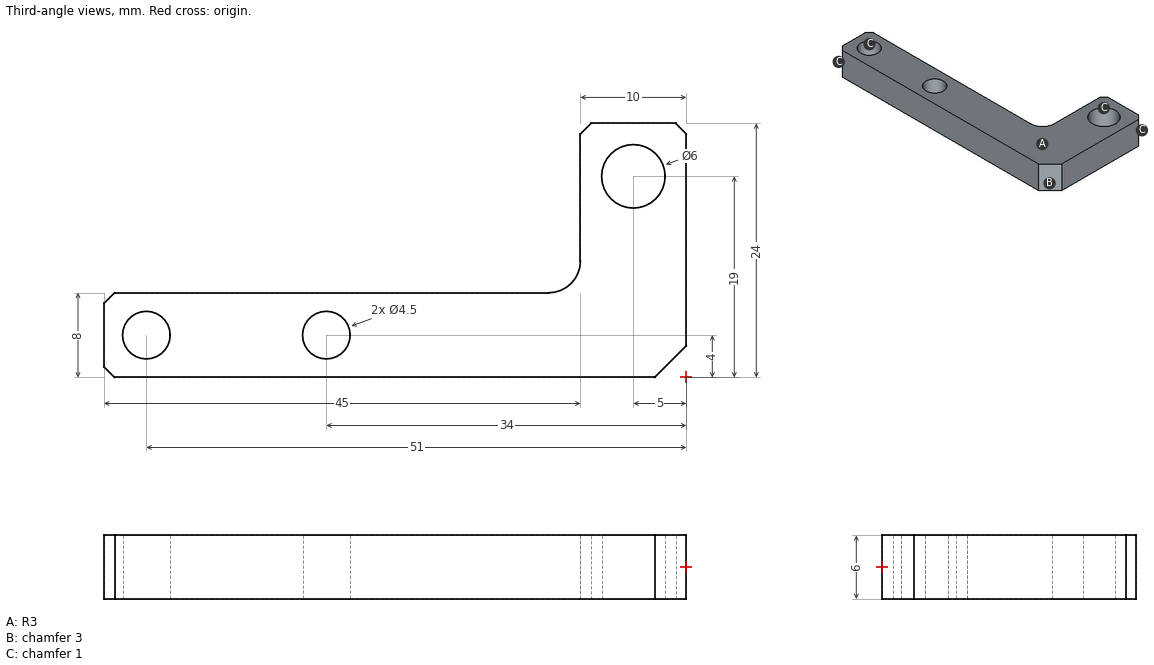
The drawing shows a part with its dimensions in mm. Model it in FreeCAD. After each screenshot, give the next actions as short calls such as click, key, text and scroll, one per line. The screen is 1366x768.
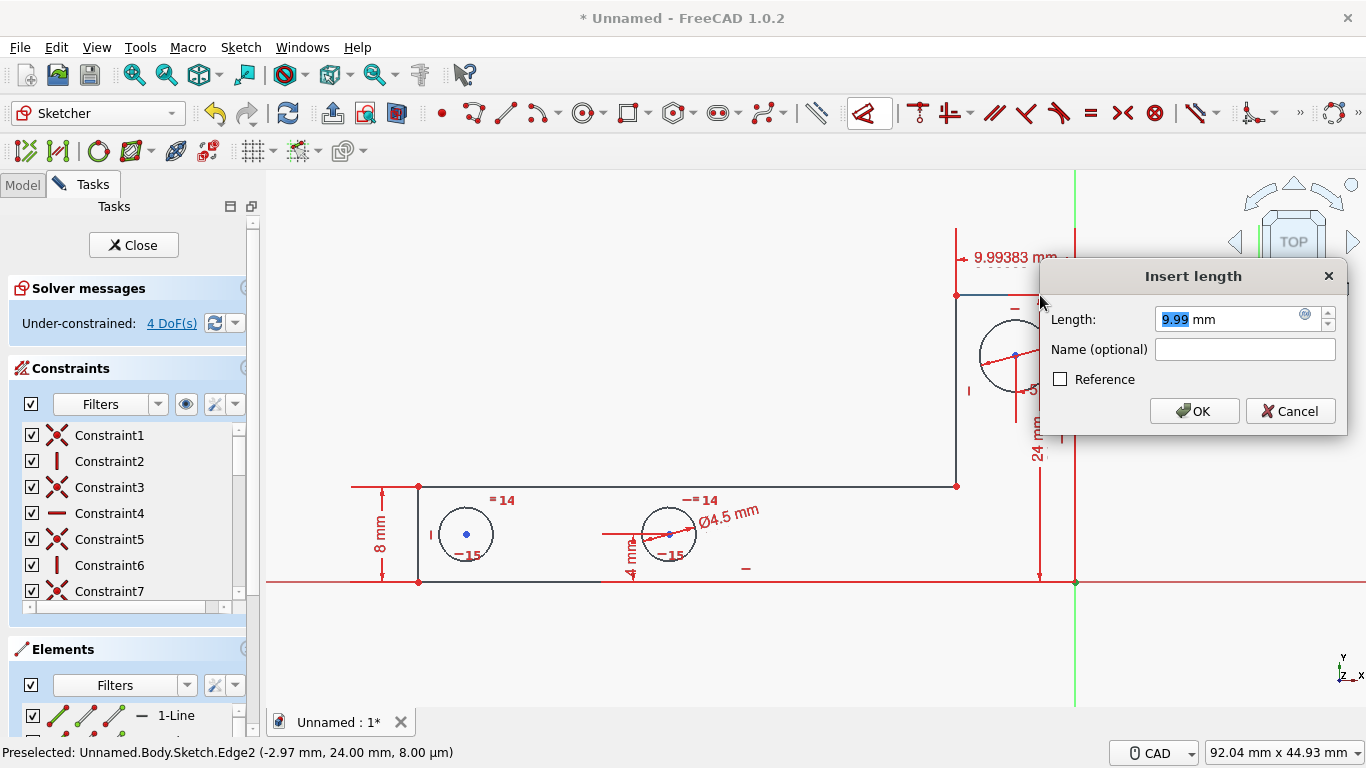
text(10)
key(Return)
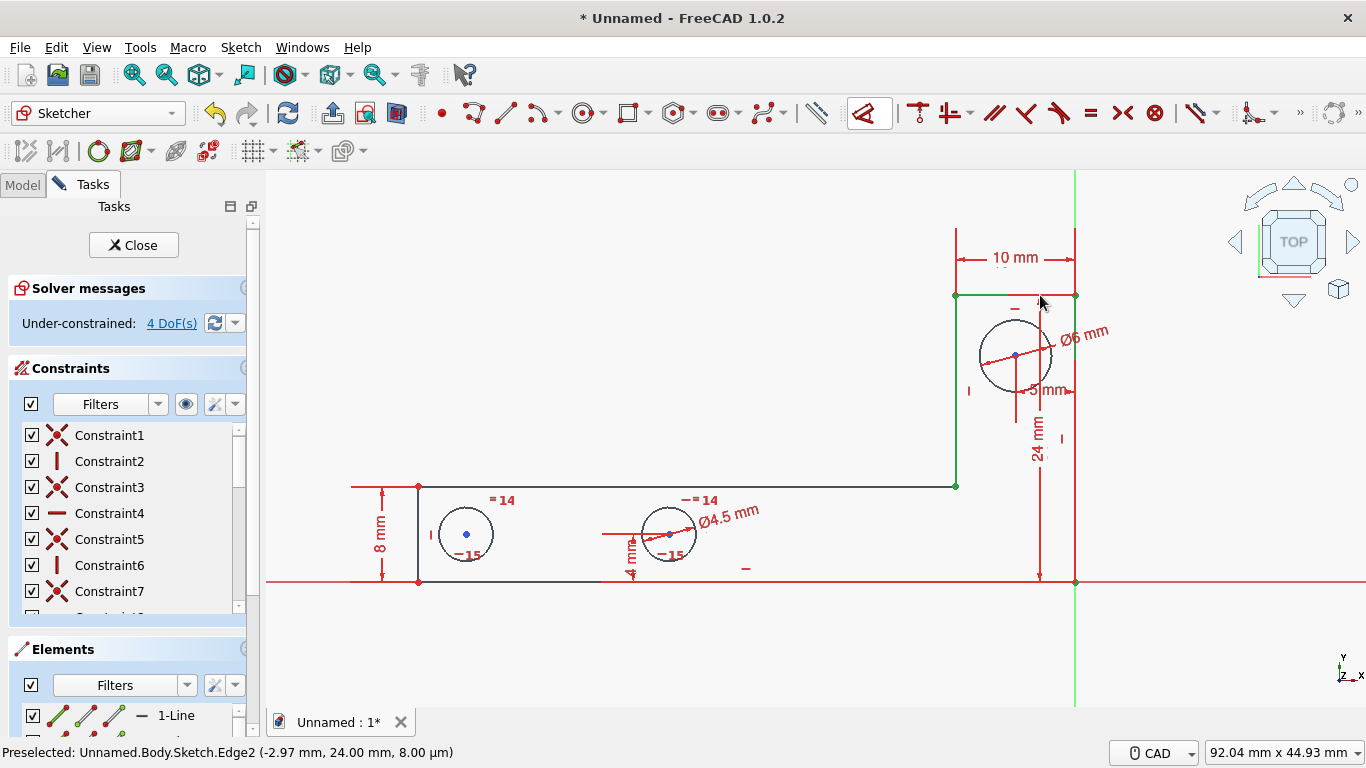
click(795, 487)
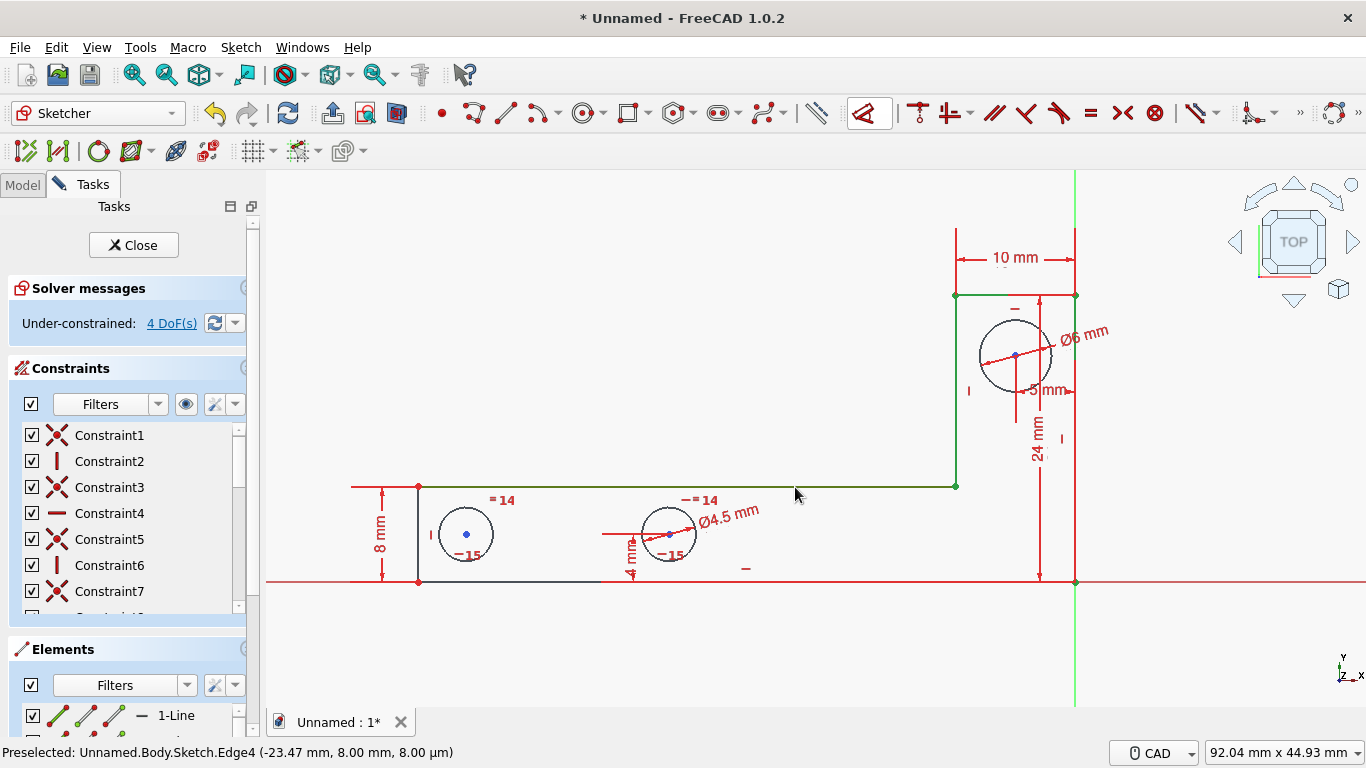
key(l)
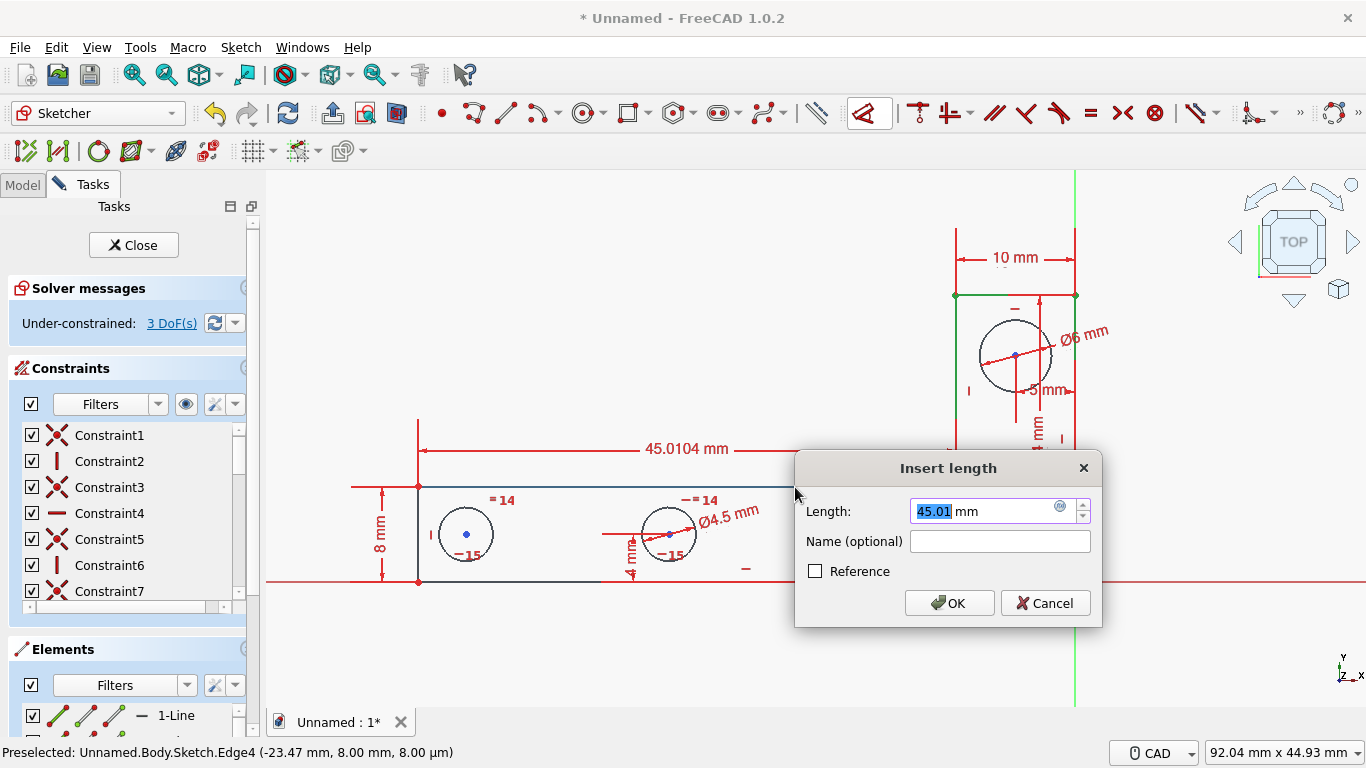
text(45)
key(Return)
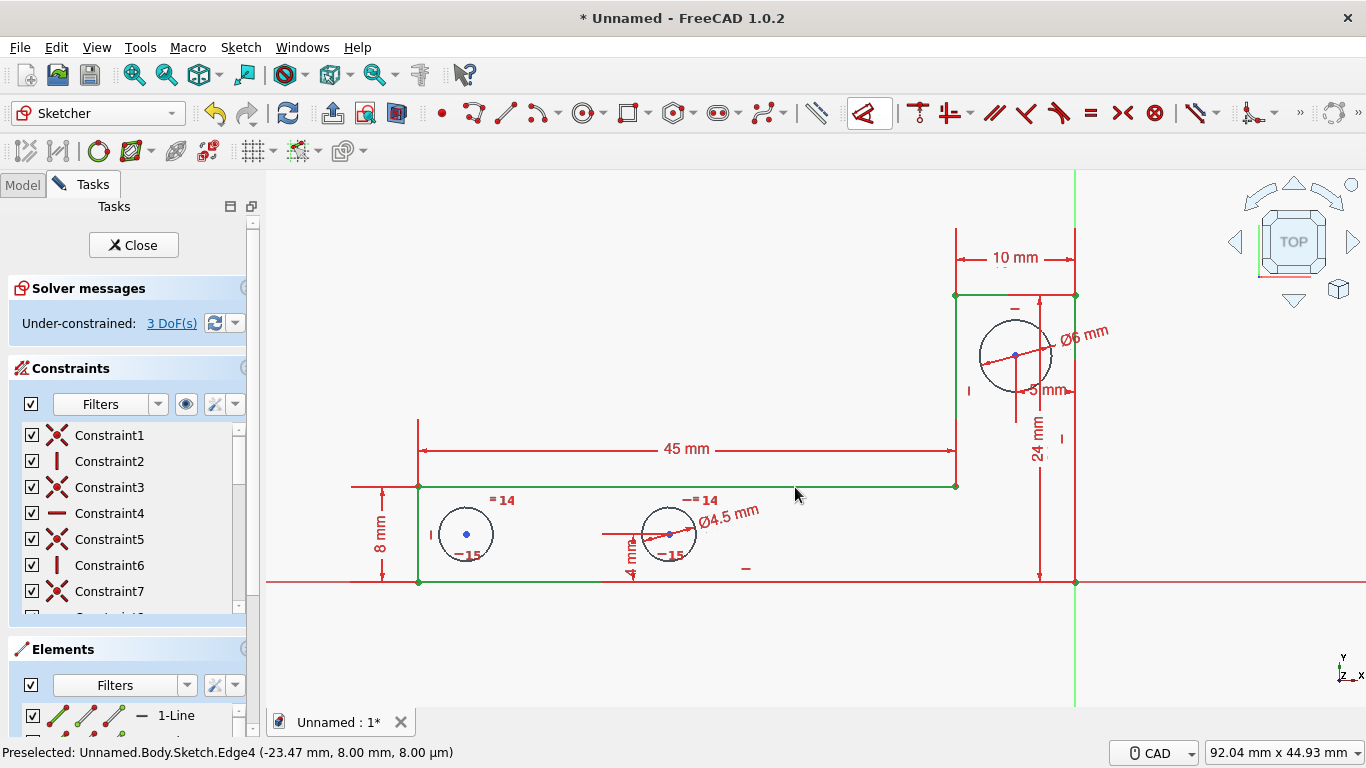
click(669, 534)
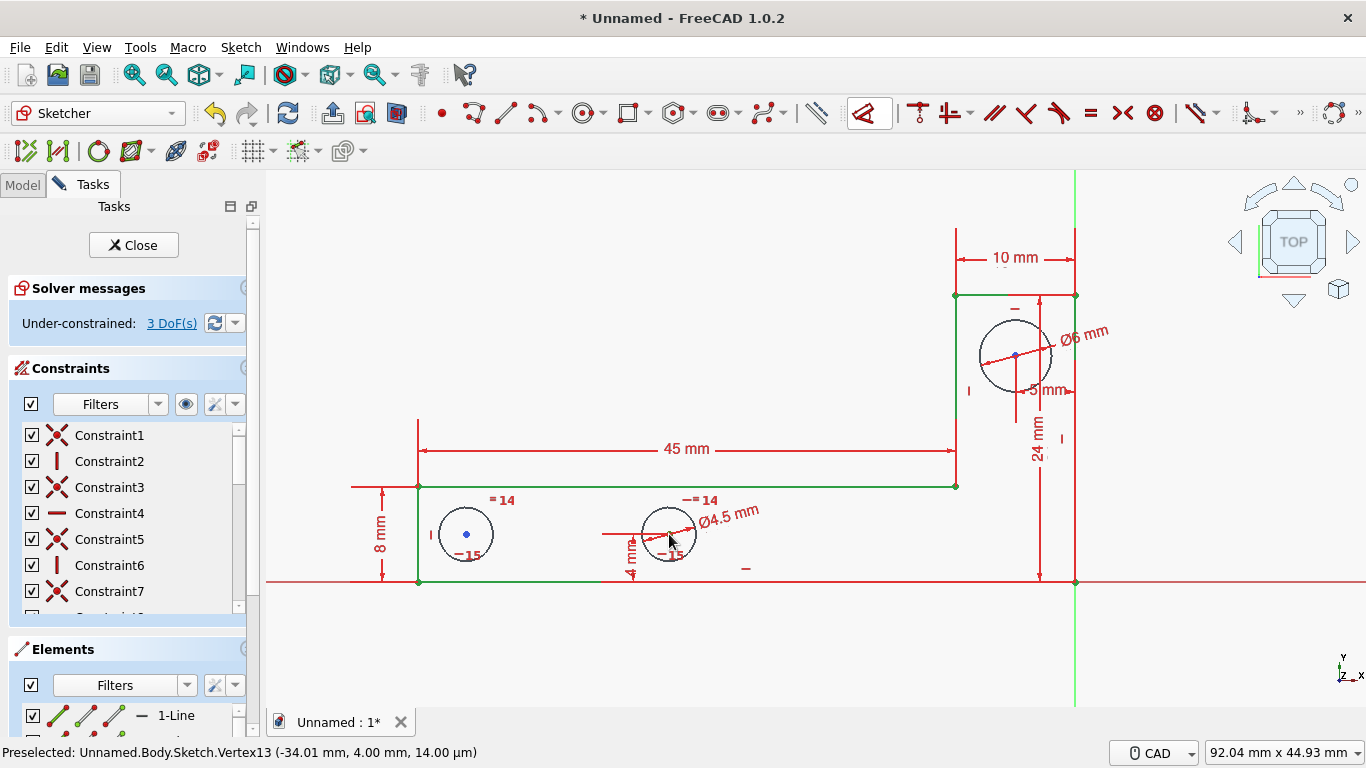
key(l)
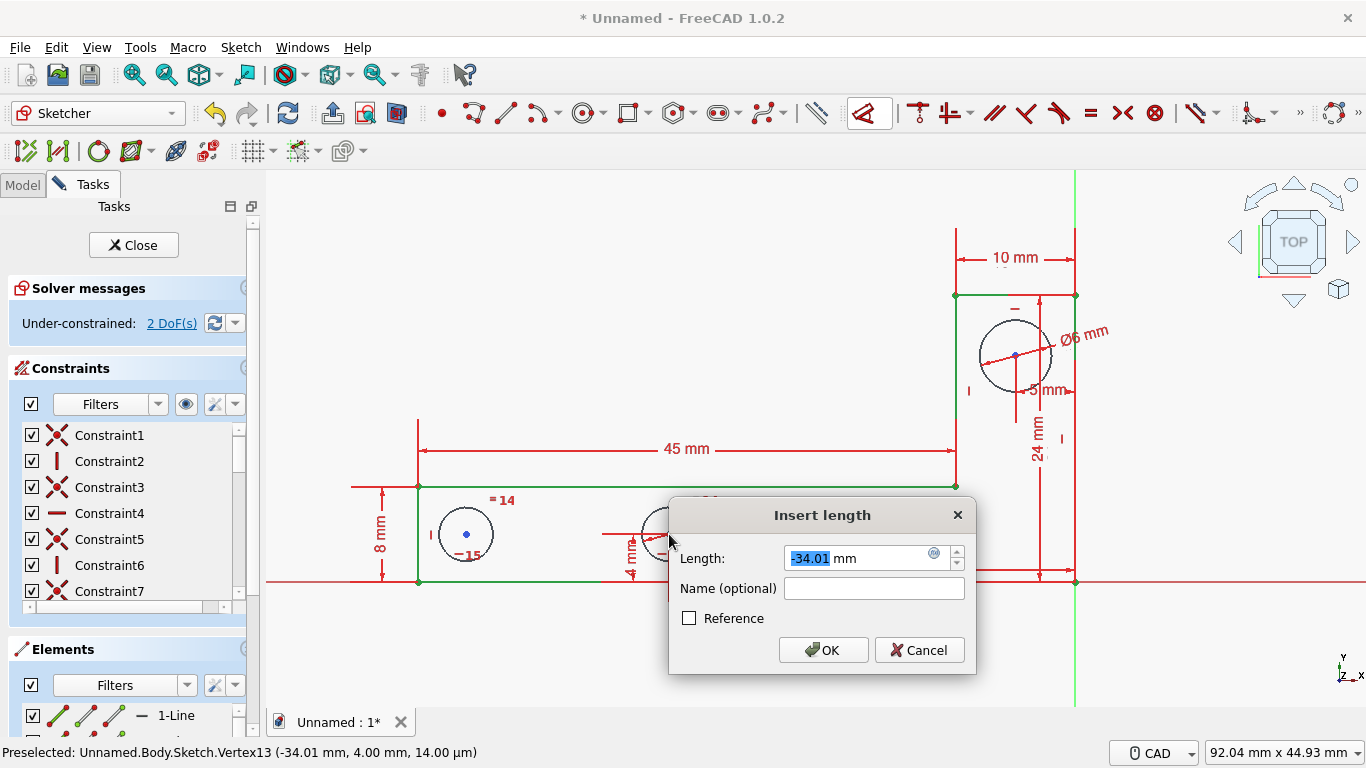
text(-34)
key(Return)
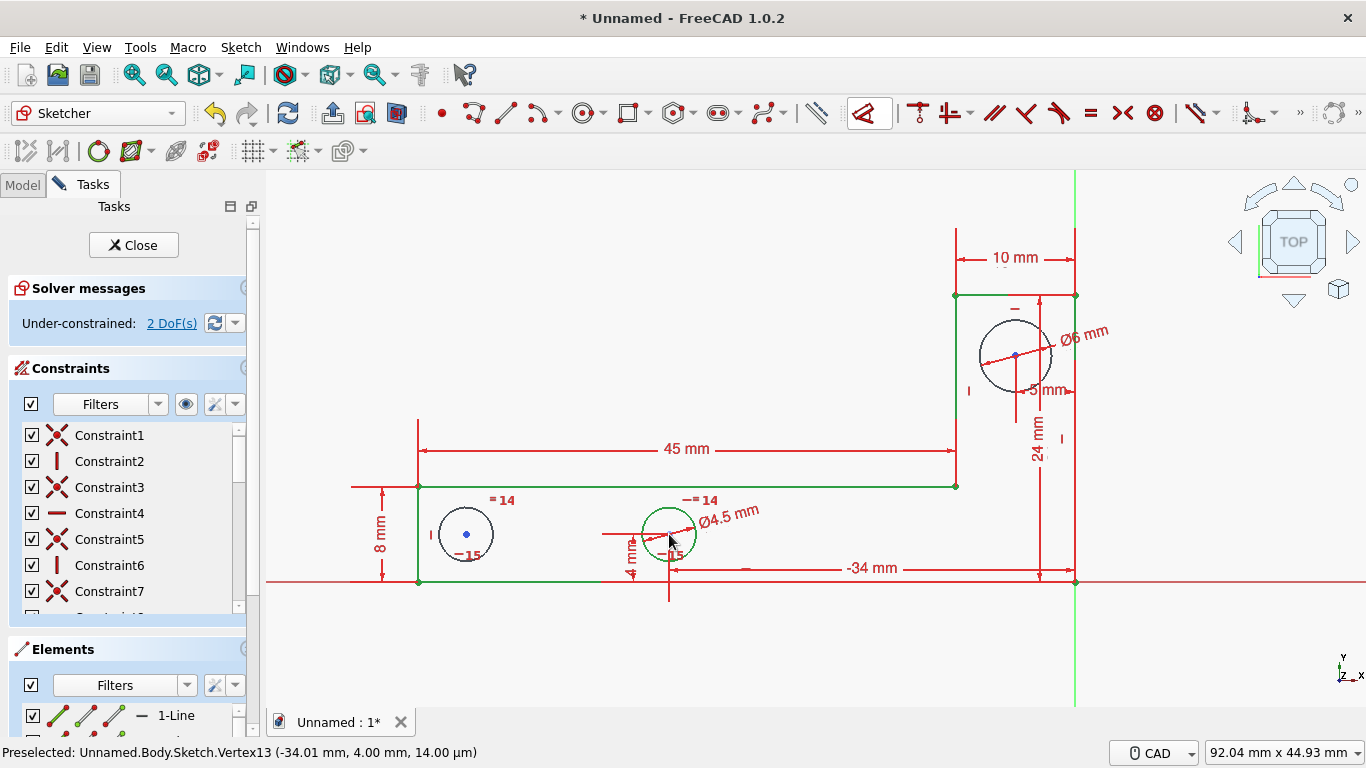
click(466, 534)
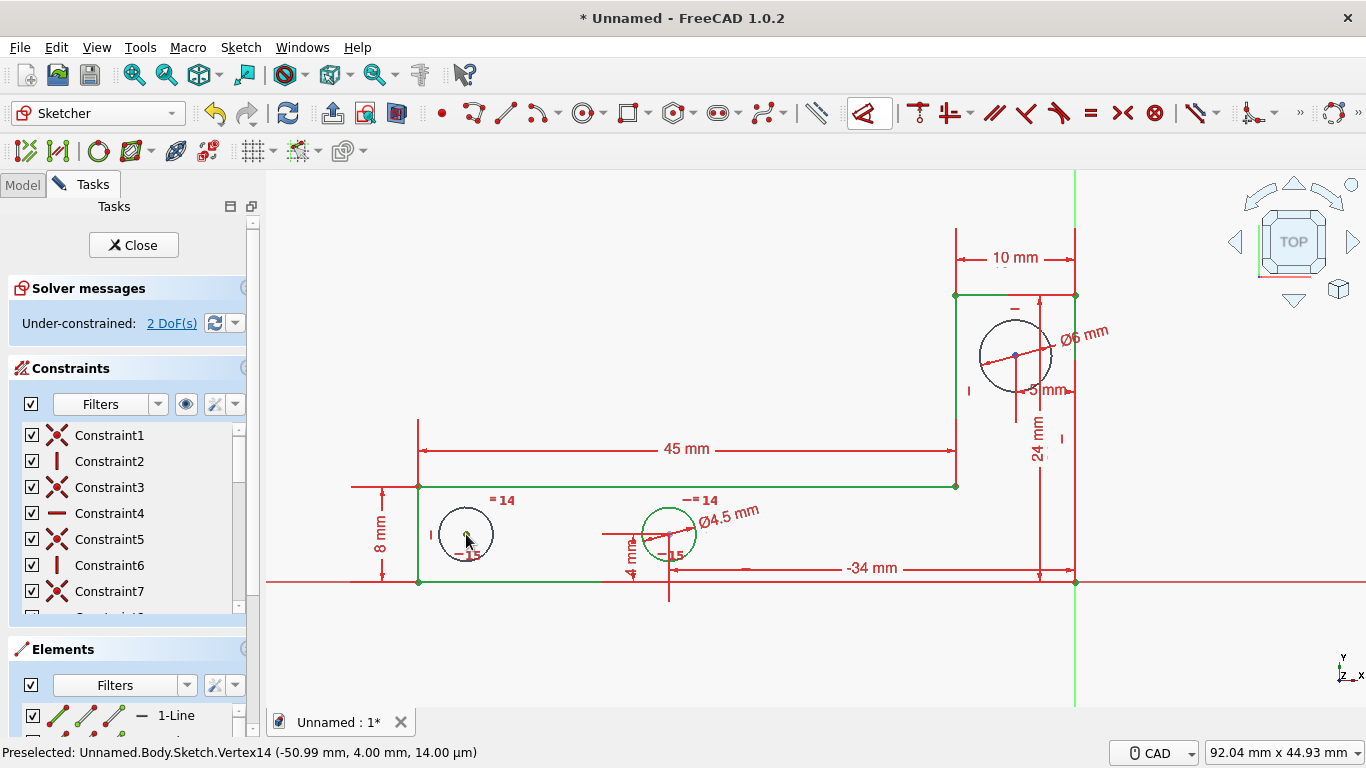
key(l)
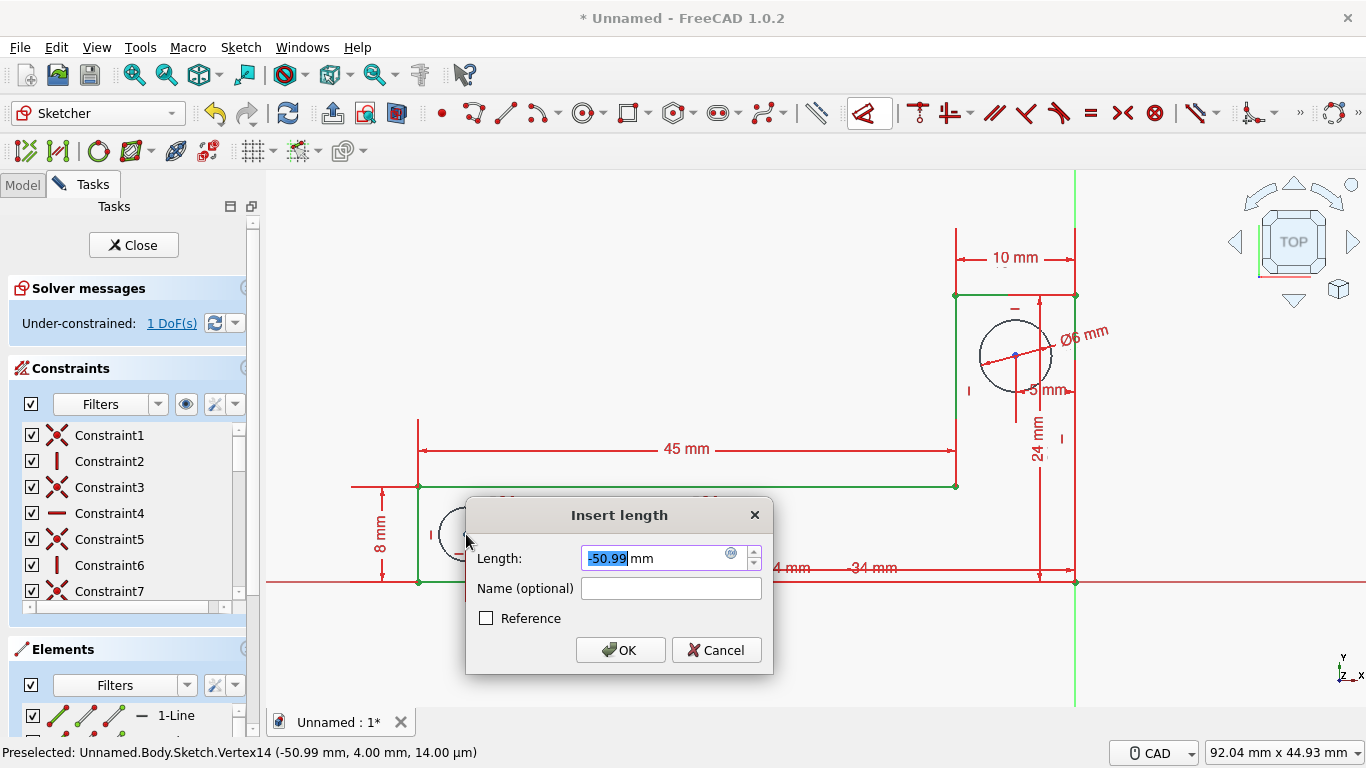
text(-51)
key(Return)